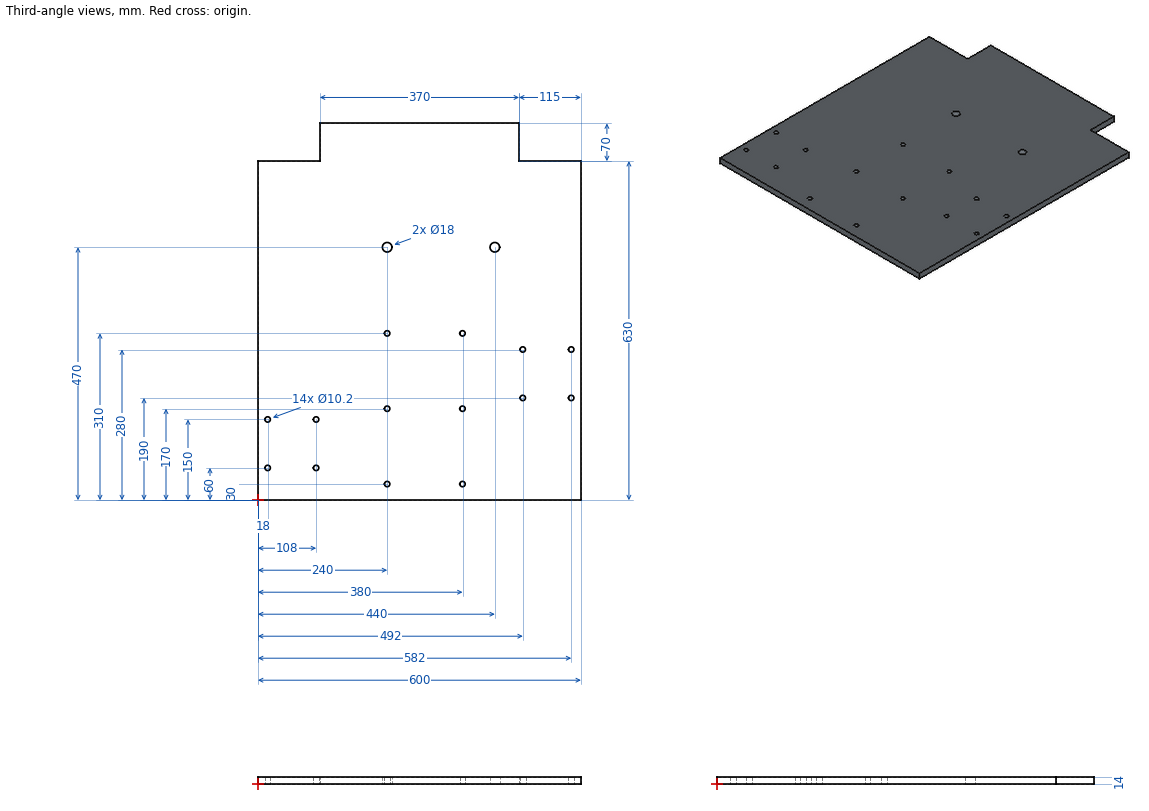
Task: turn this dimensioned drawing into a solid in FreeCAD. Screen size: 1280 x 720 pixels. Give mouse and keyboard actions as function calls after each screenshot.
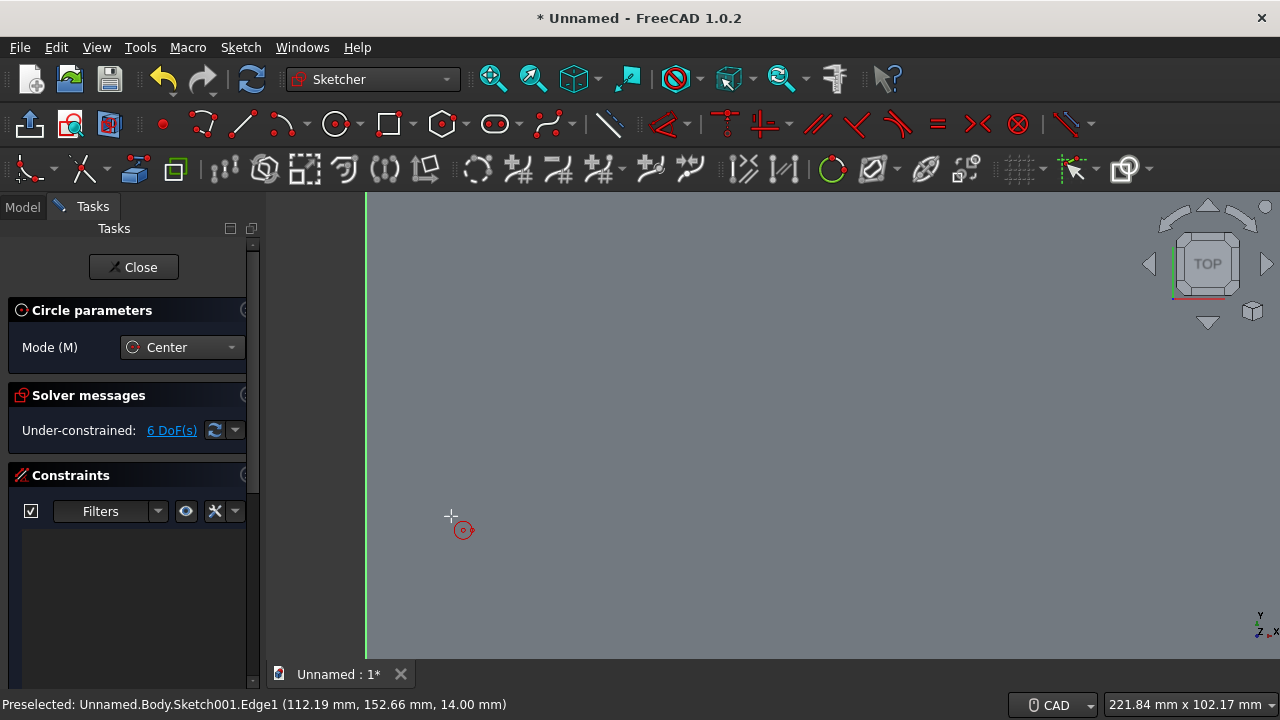
scroll(451, 516, down, 8)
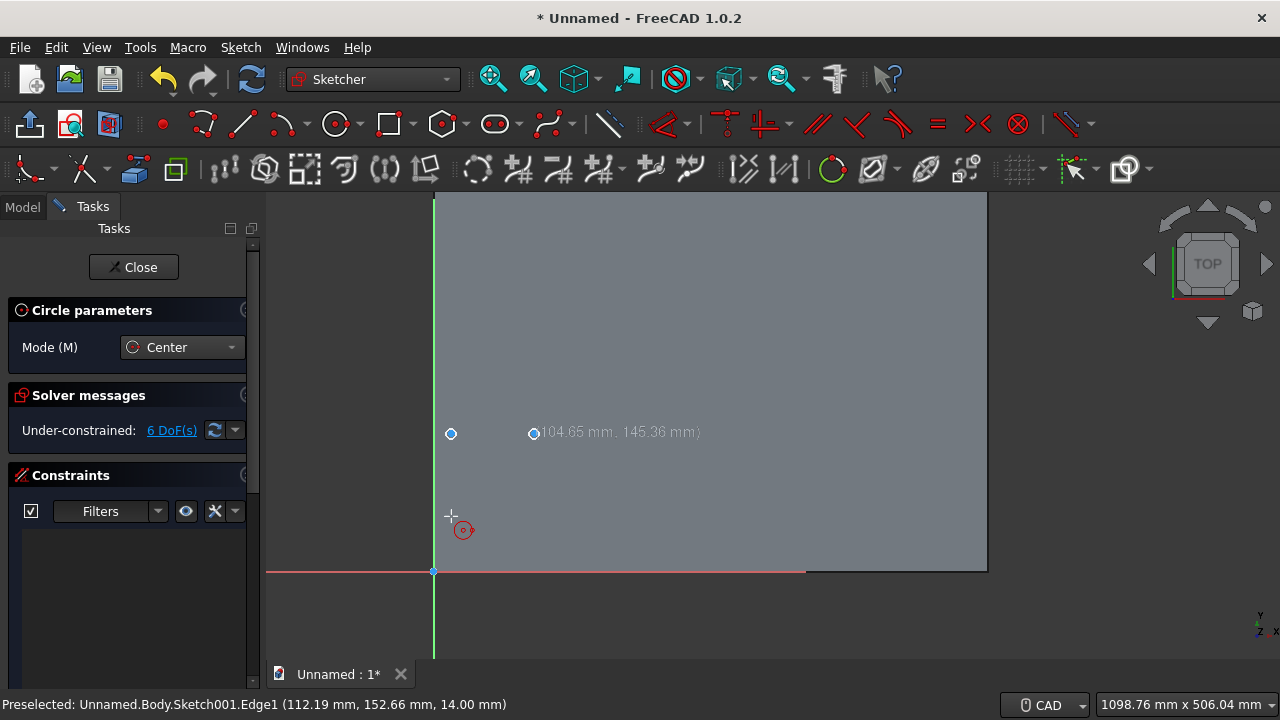
click(451, 516)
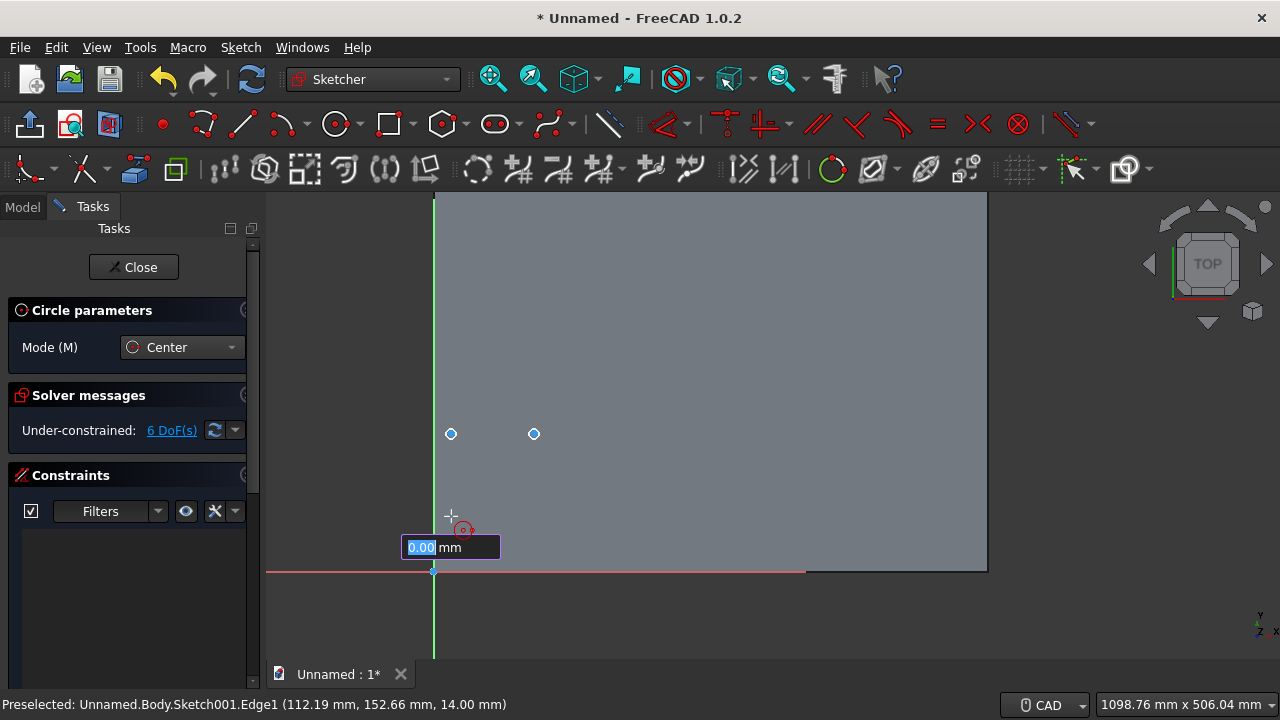
scroll(454, 513, up, 7)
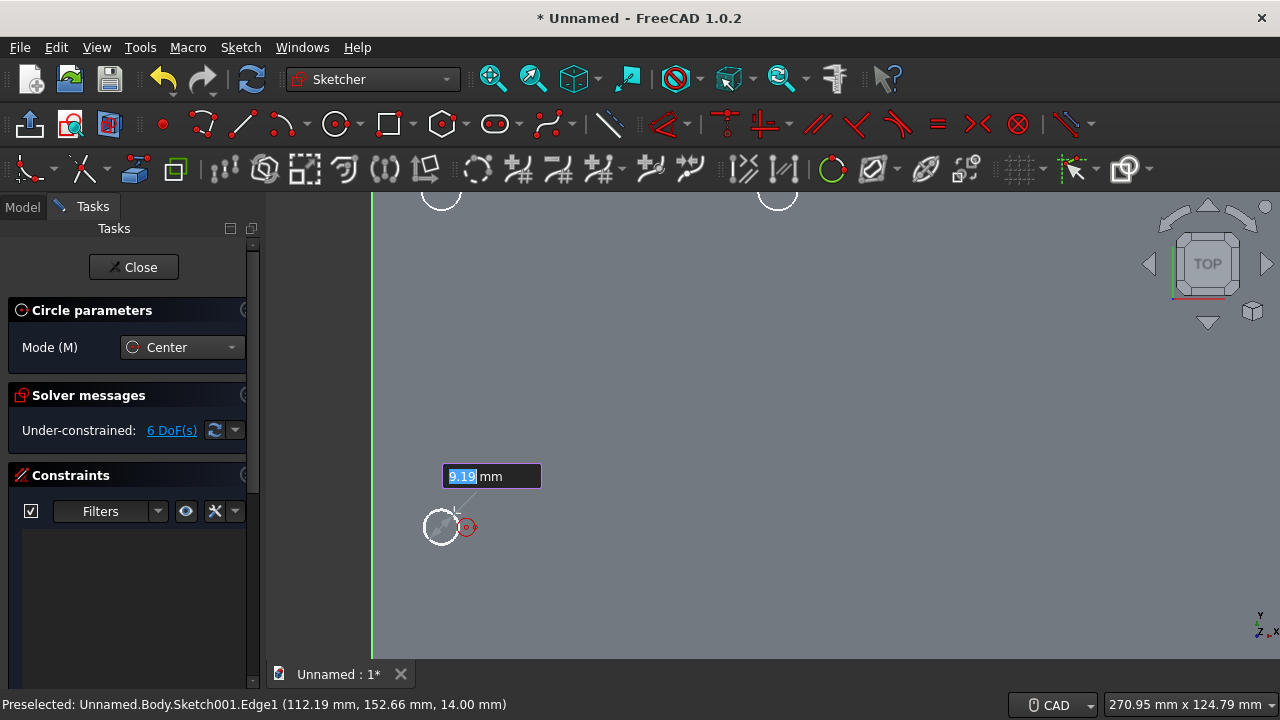
click(453, 510)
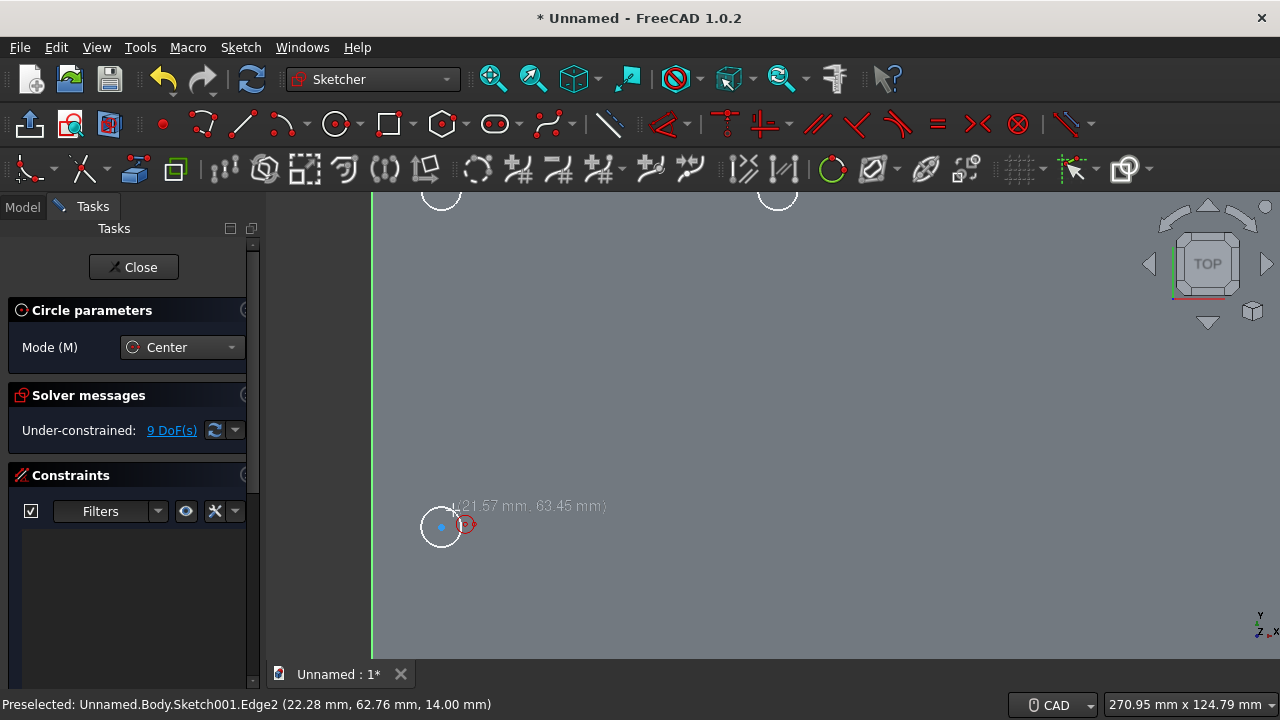
scroll(454, 513, down, 7)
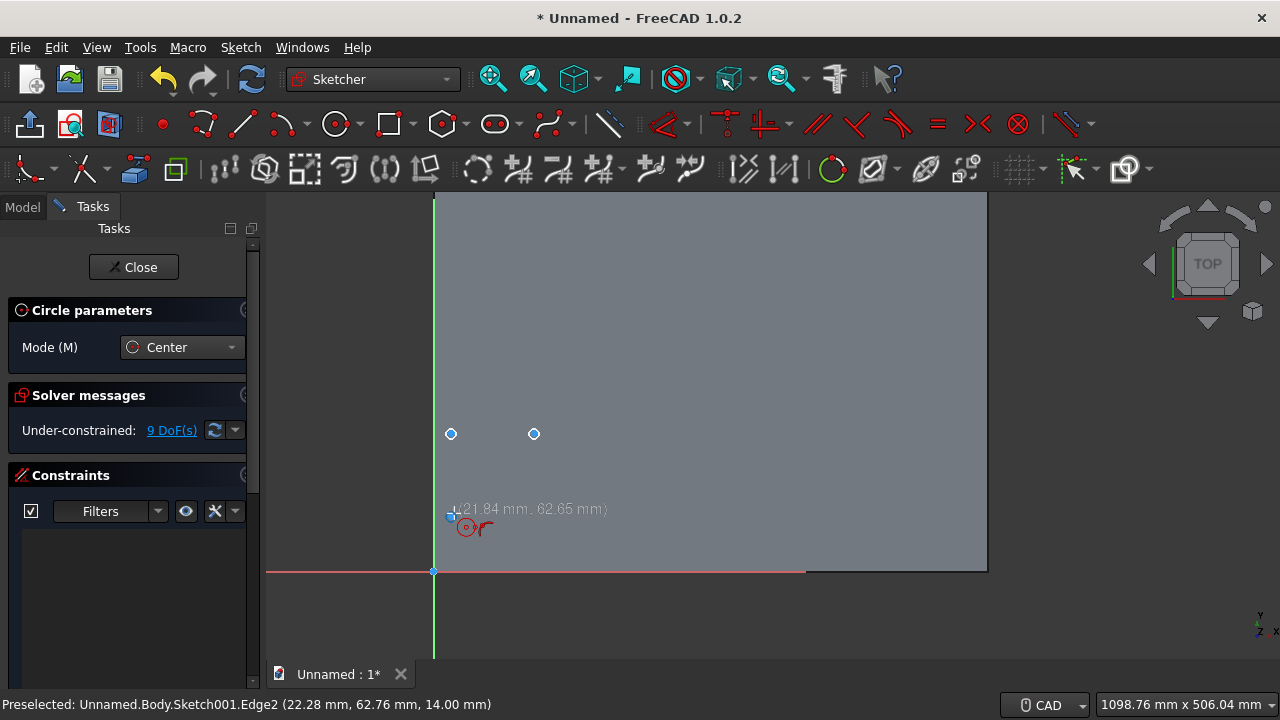
click(534, 516)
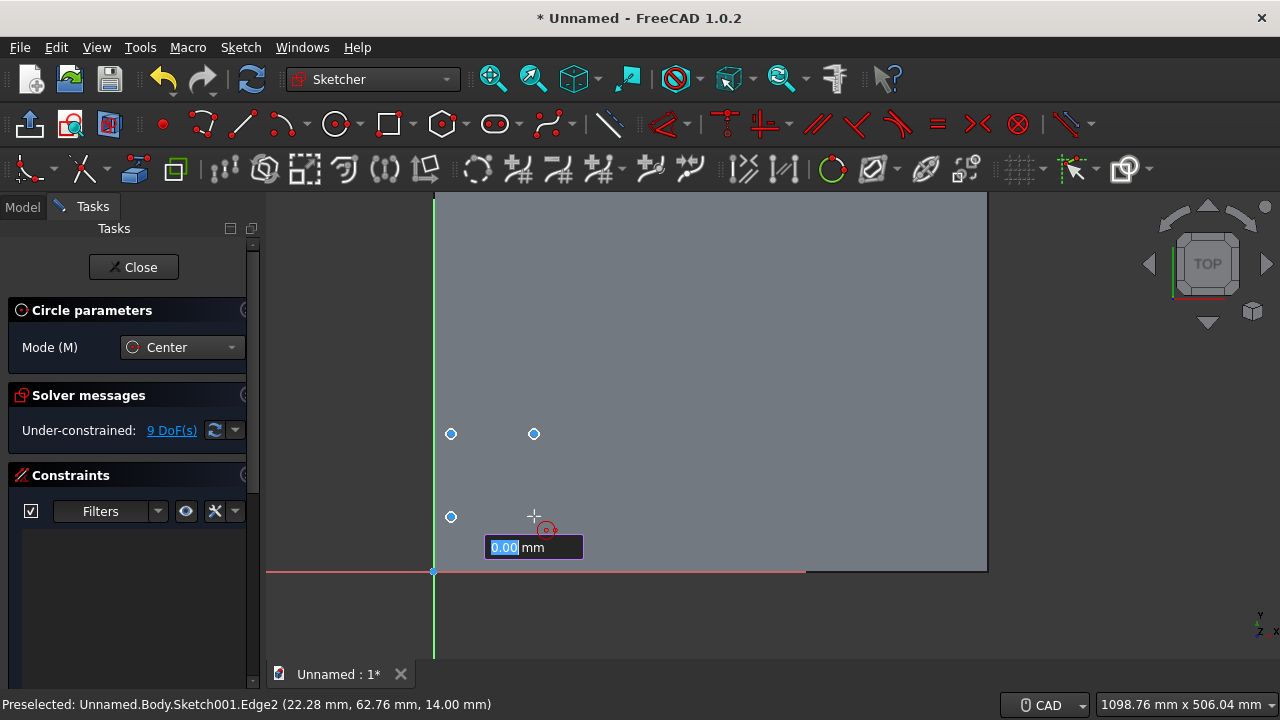
scroll(537, 513, up, 7)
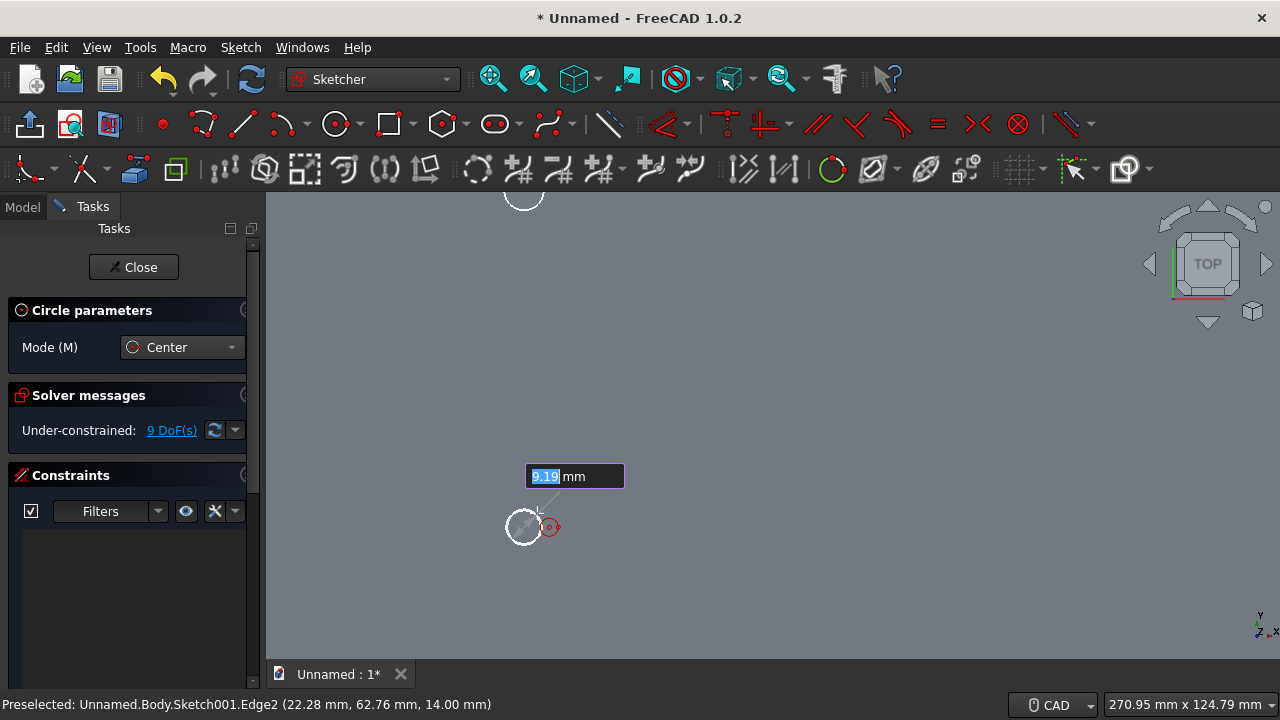
click(536, 510)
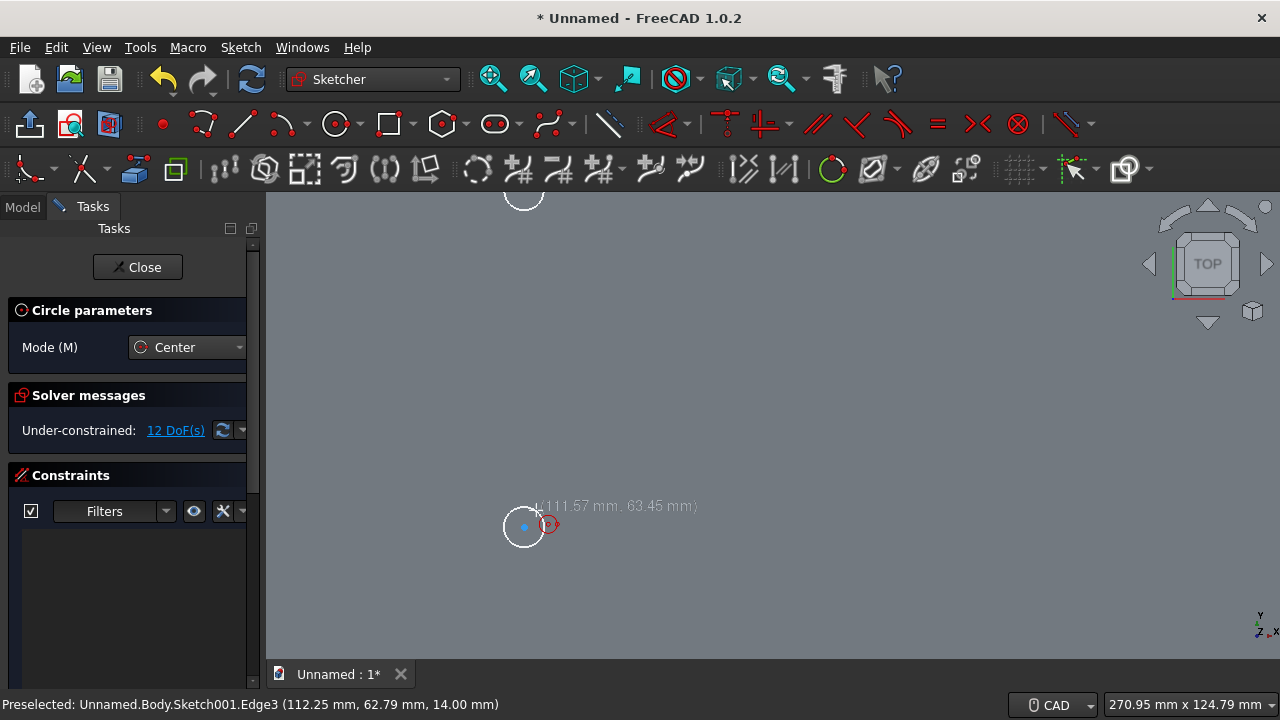
scroll(537, 513, down, 7)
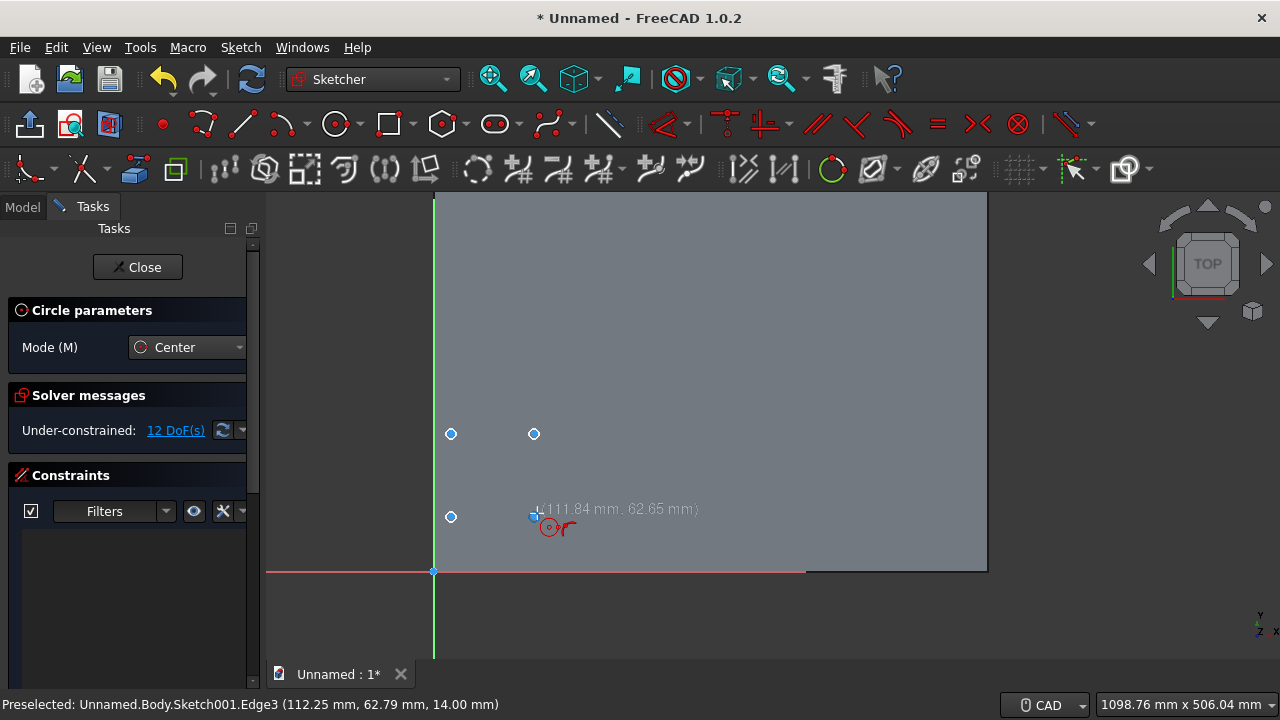
scroll(888, 313, up, 8)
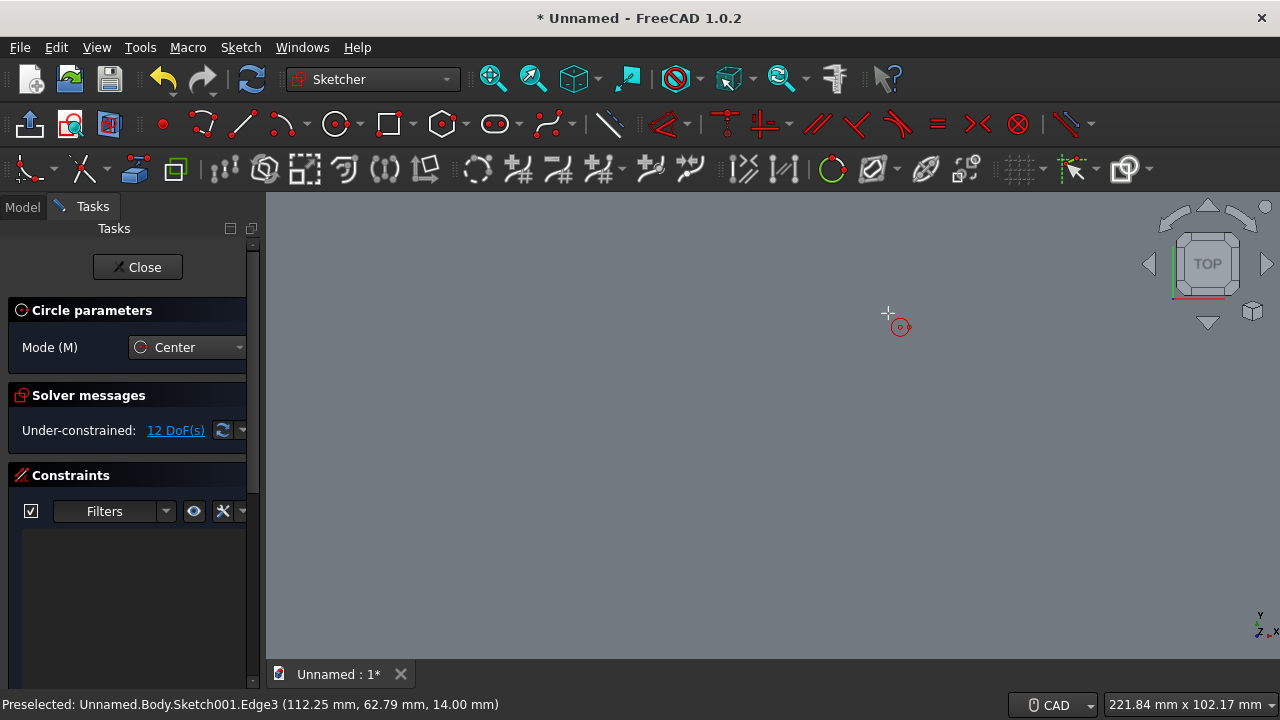
scroll(888, 312, down, 8)